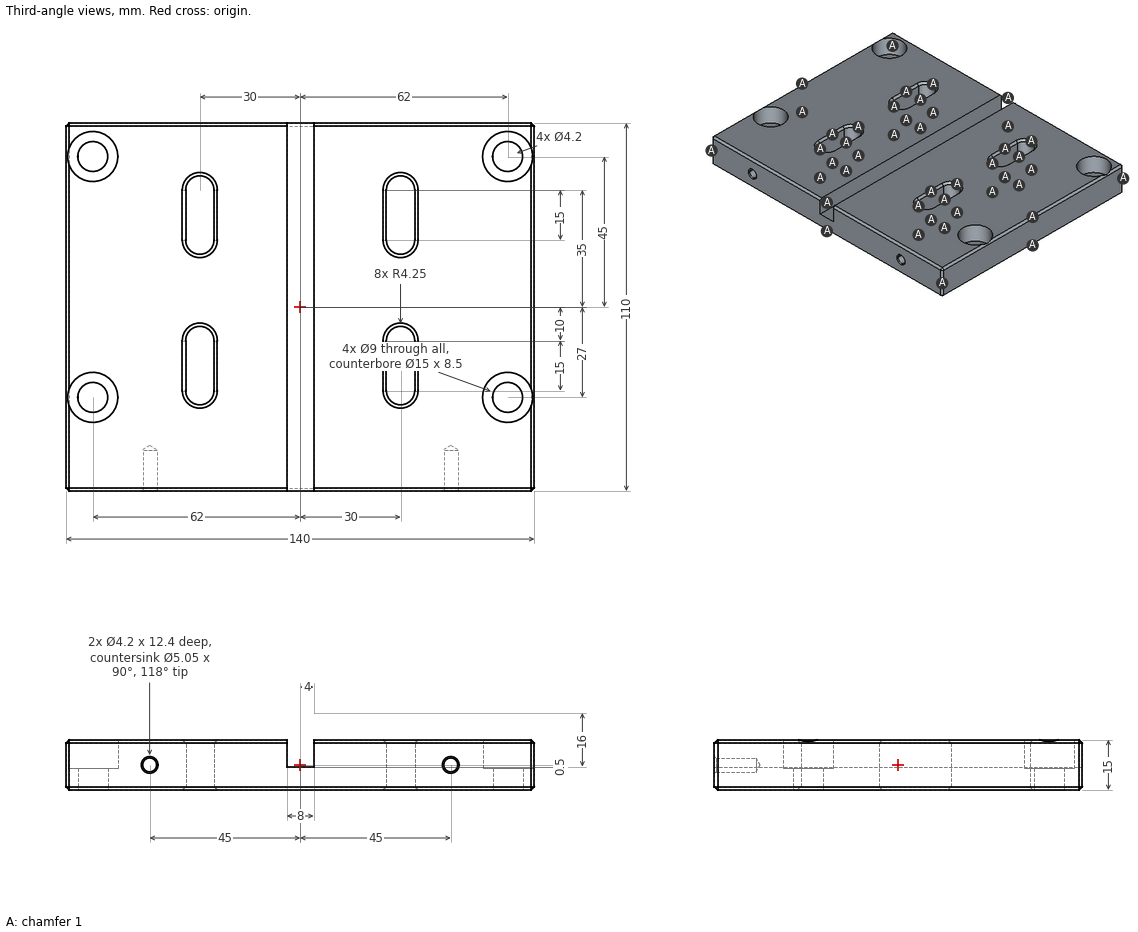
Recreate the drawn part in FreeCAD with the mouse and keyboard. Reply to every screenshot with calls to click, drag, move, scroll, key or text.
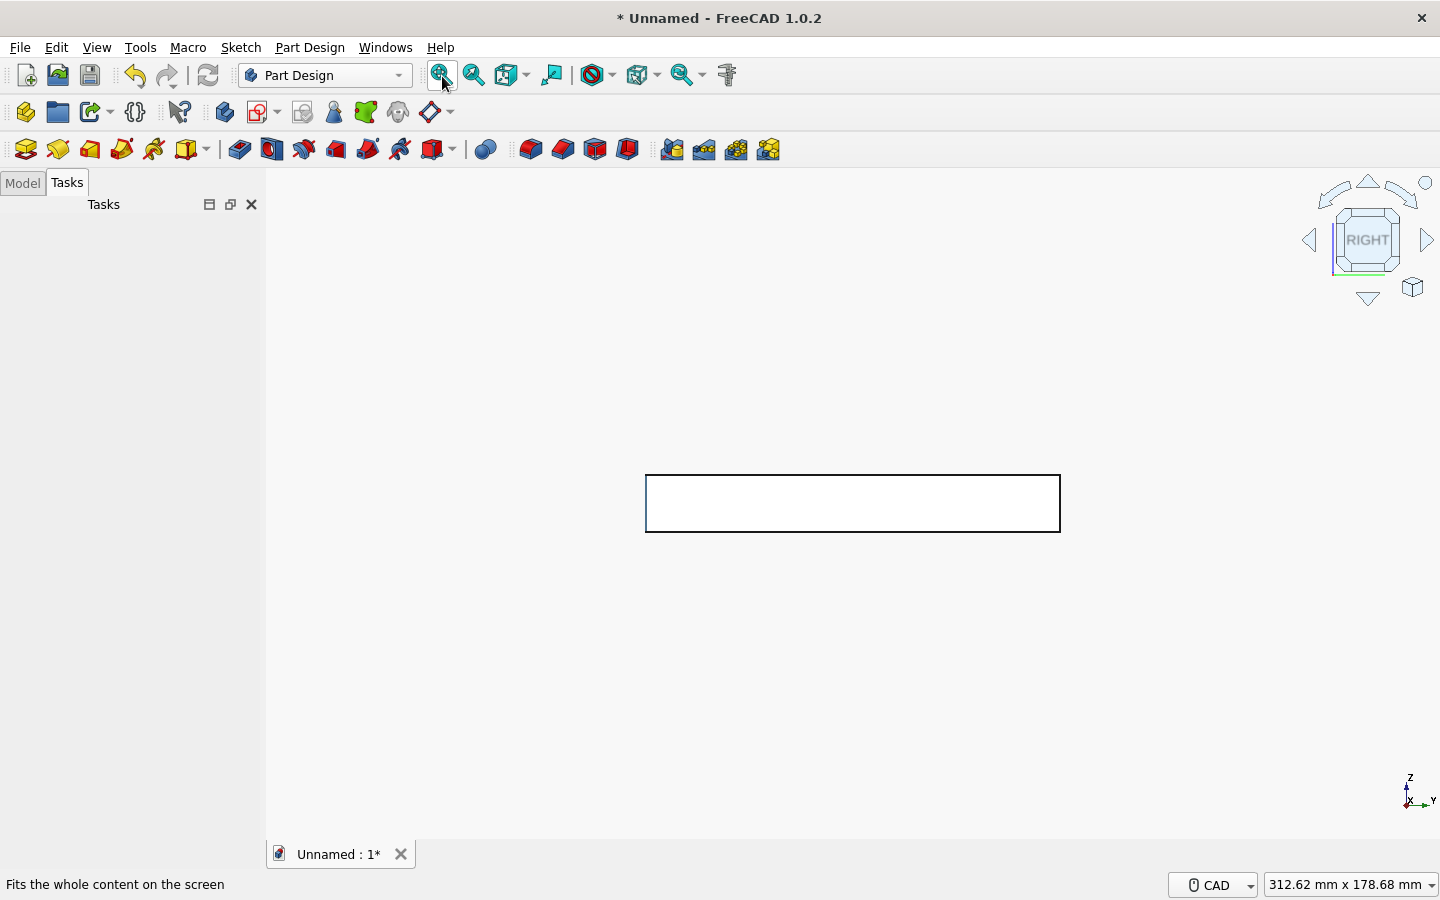
click(1060, 502, ctrl)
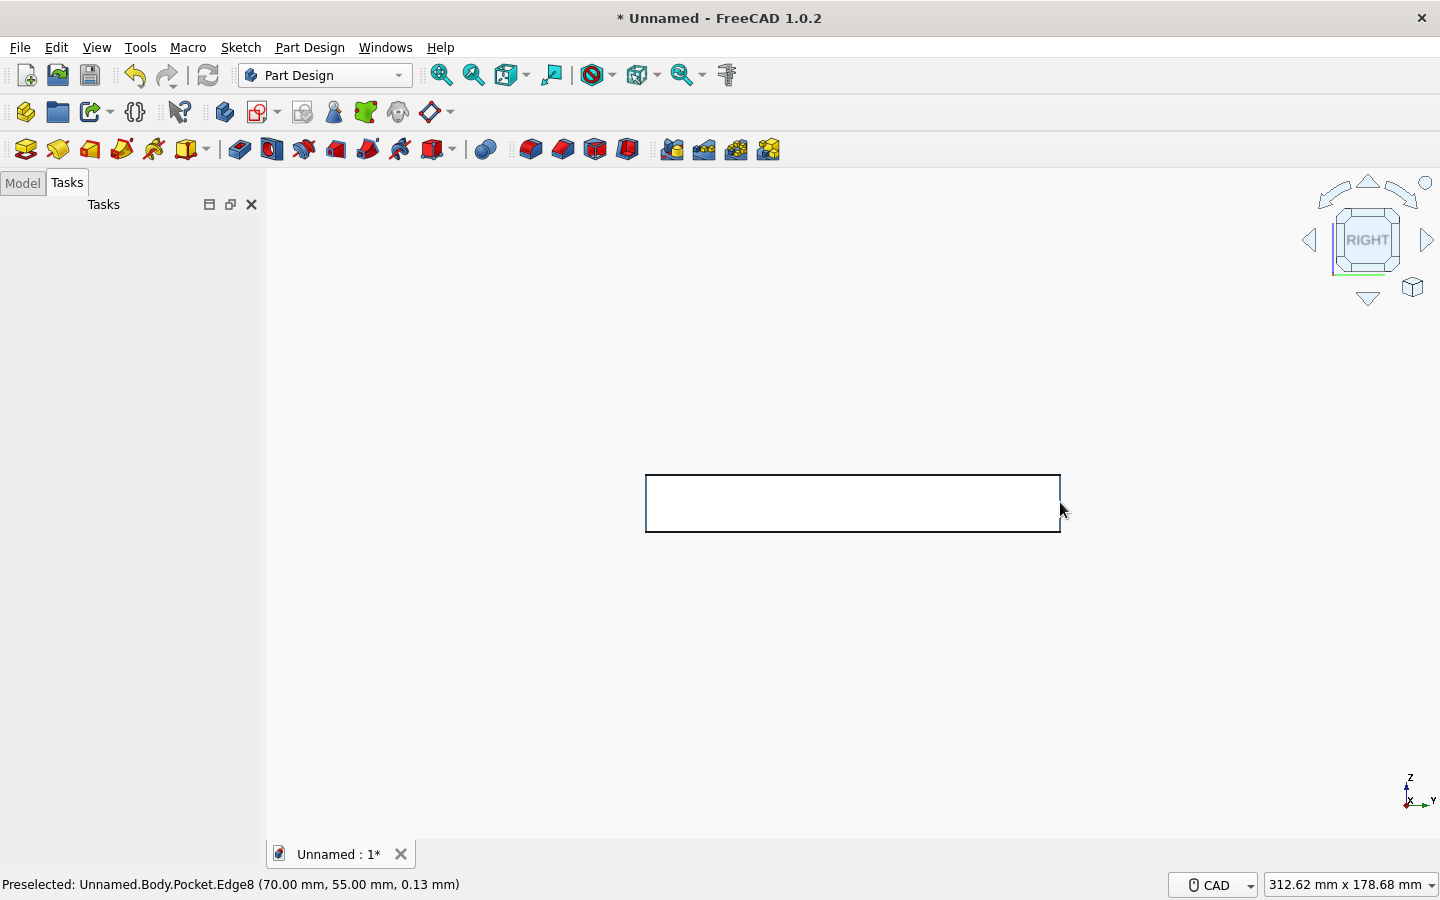
key(5)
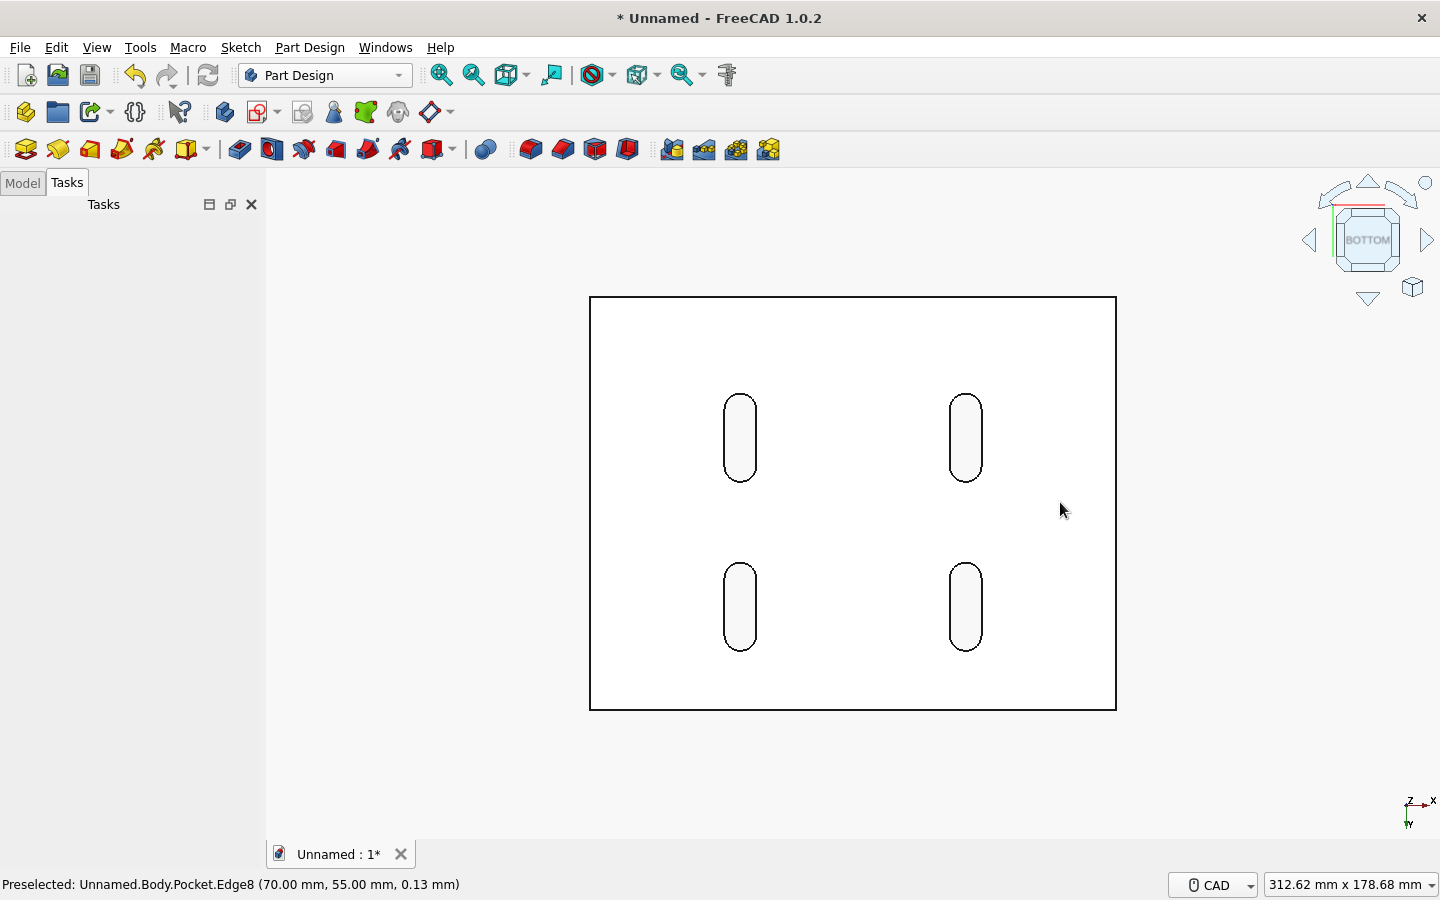
key(4)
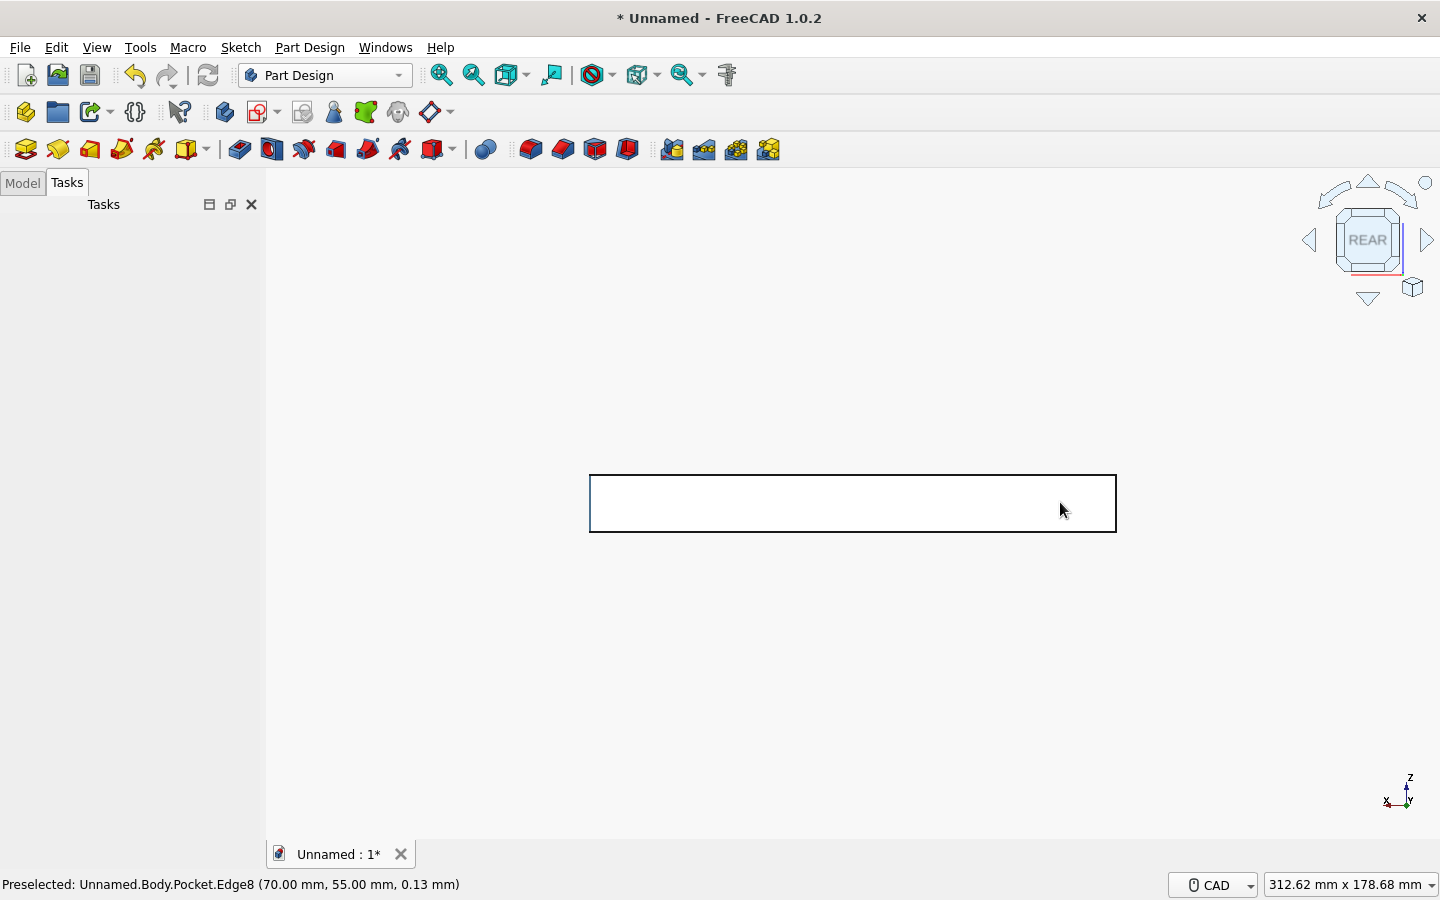
click(442, 76)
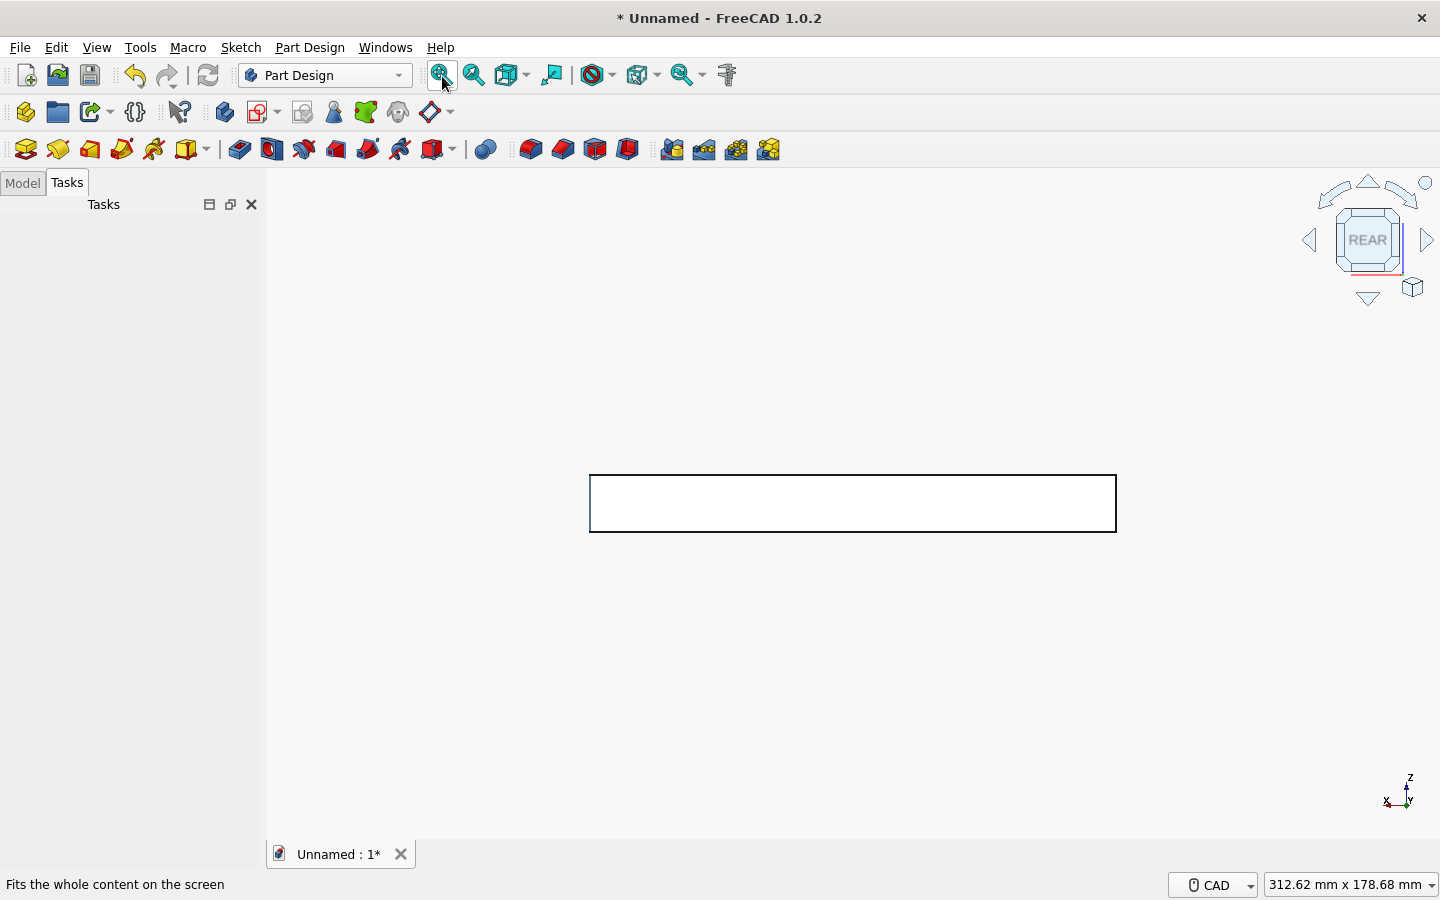
click(1116, 503, ctrl)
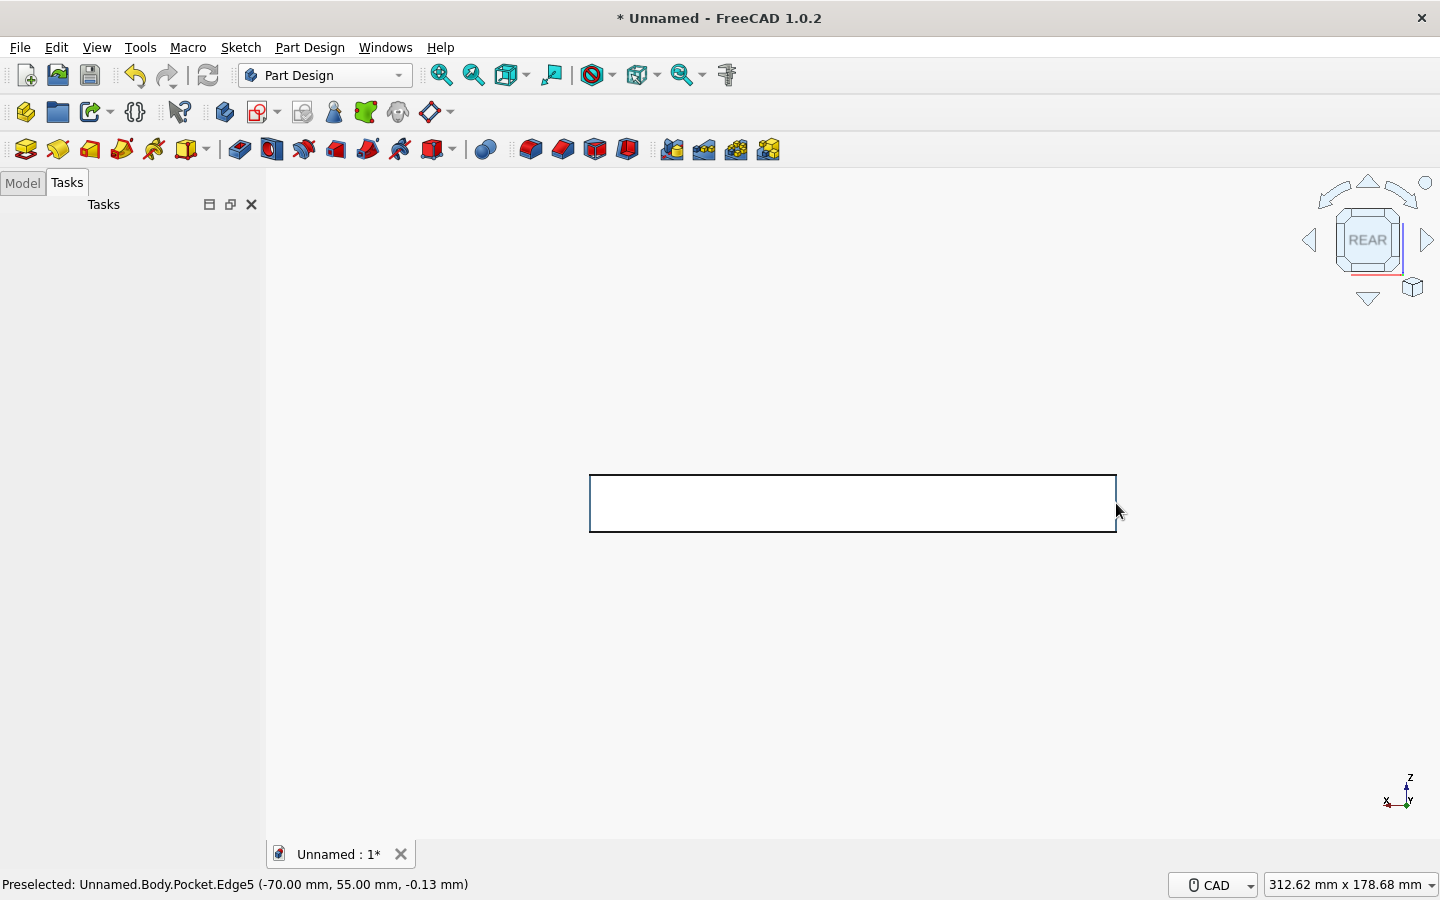
click(564, 150)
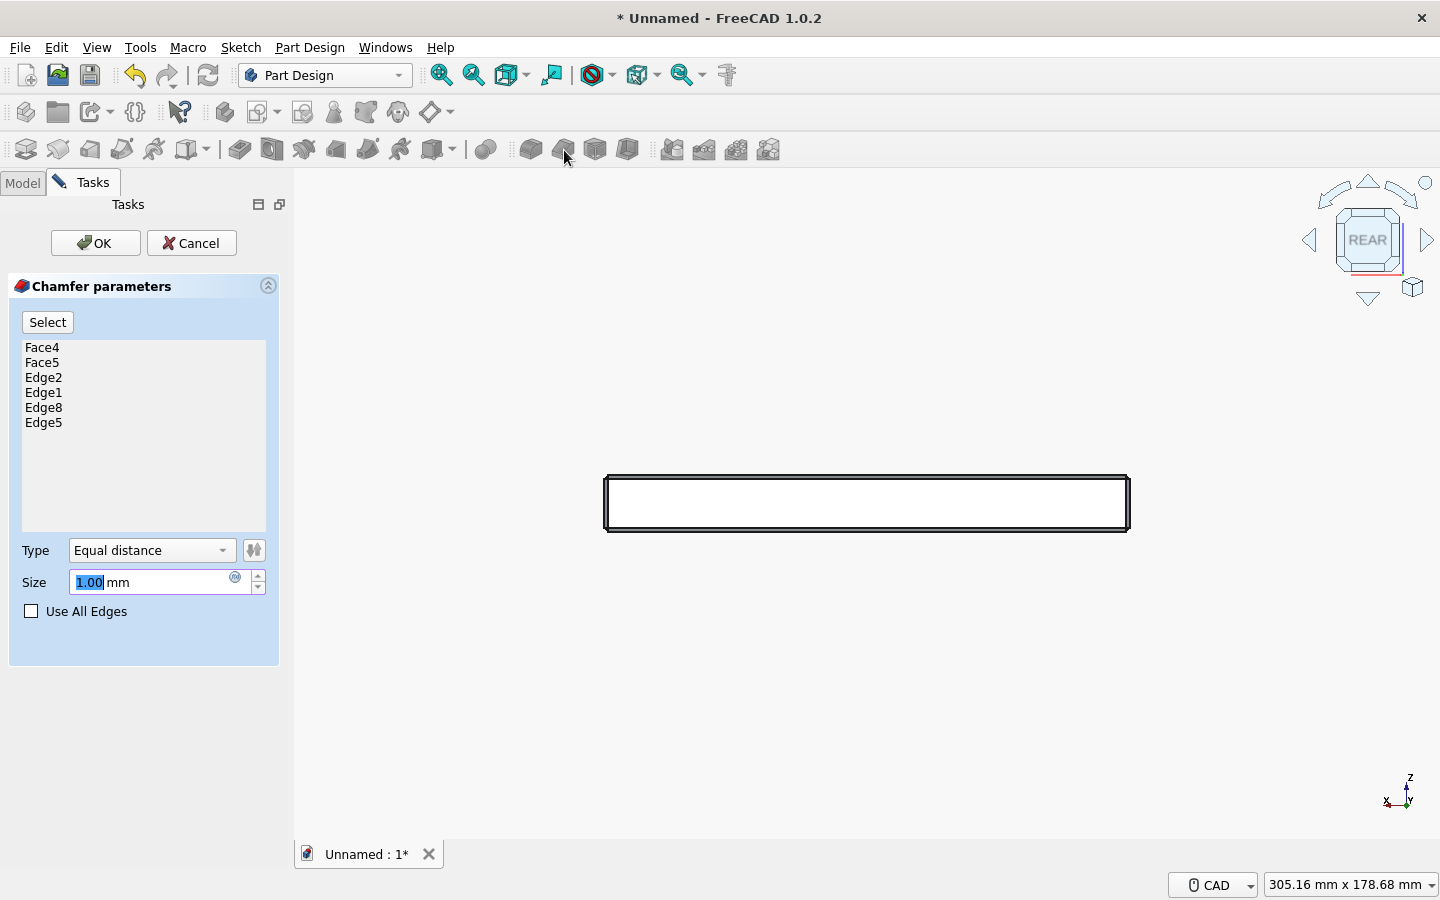
text(1)
key(Tab)